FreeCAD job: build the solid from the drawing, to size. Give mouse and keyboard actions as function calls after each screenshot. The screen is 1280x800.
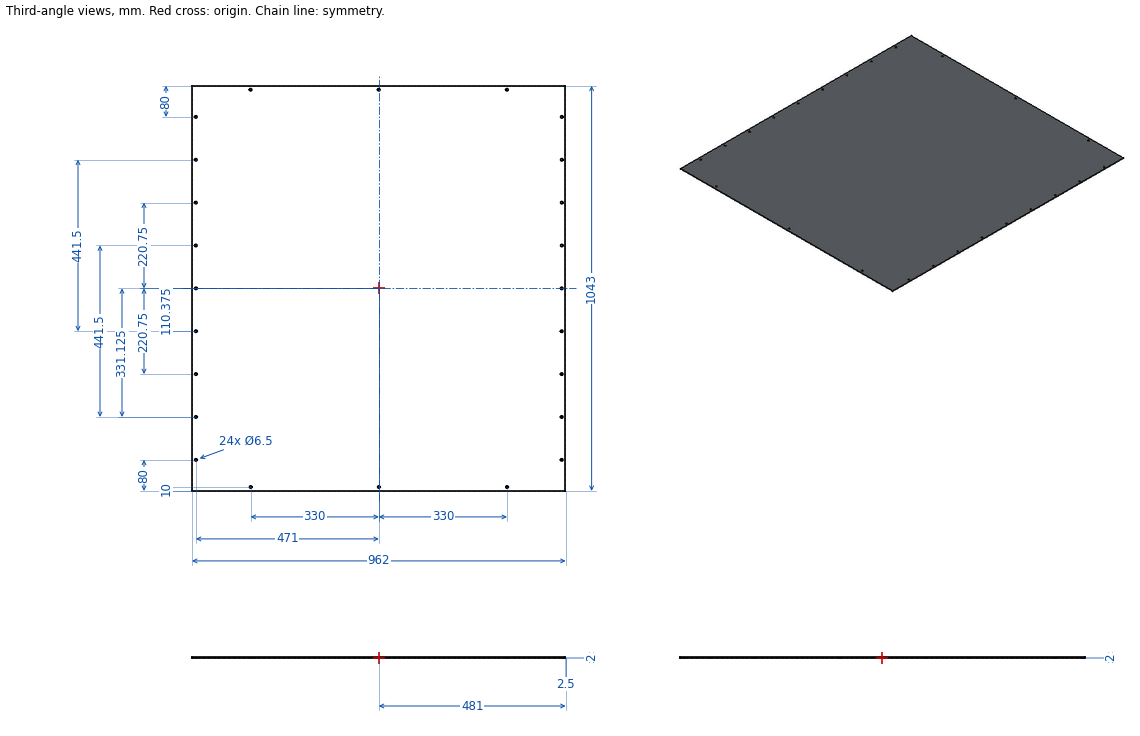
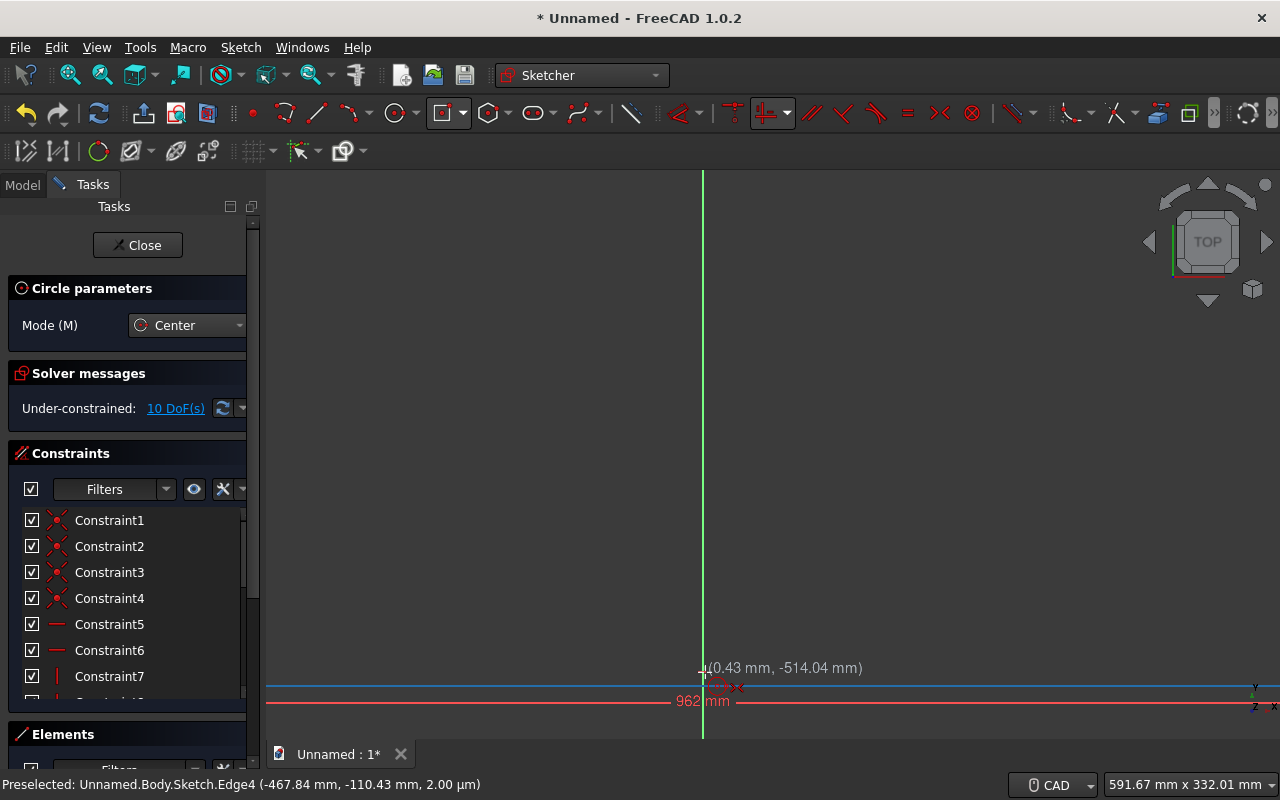
click(703, 669)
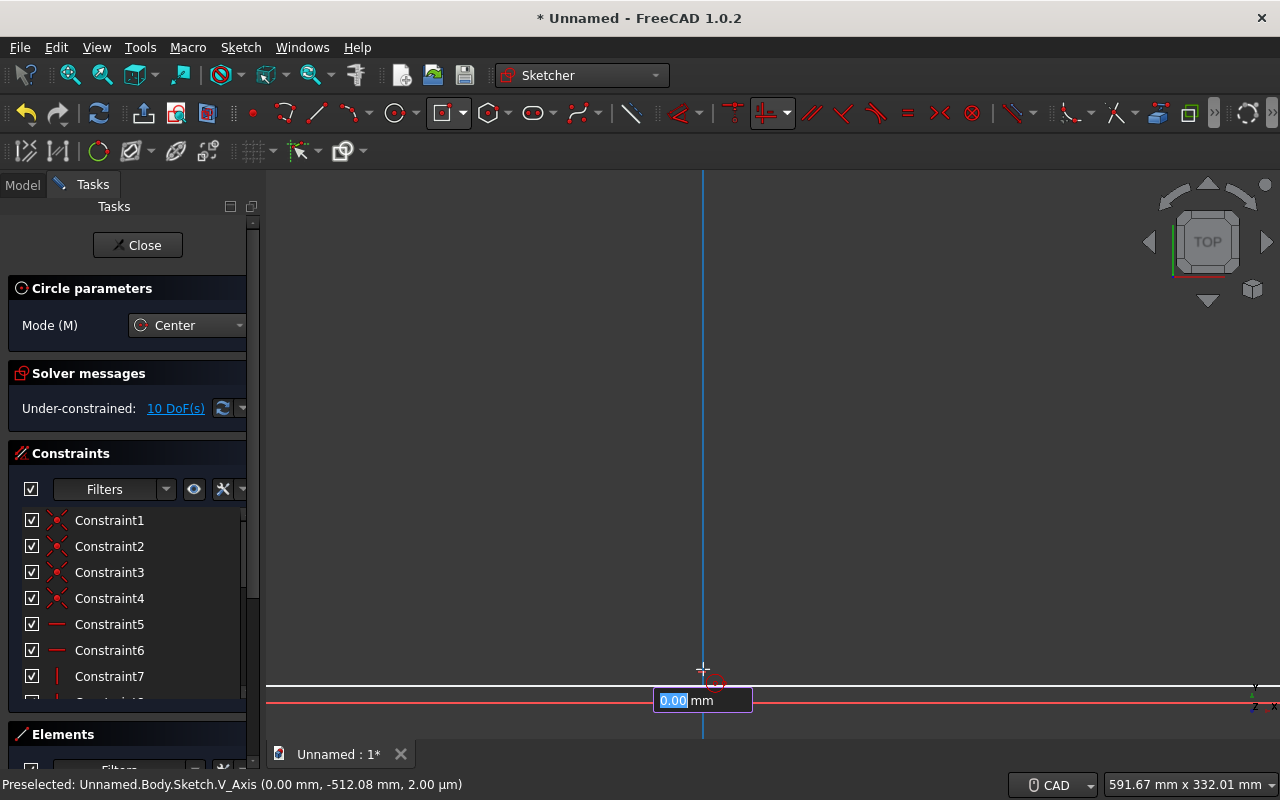
scroll(708, 667, up, 6)
move(708, 665)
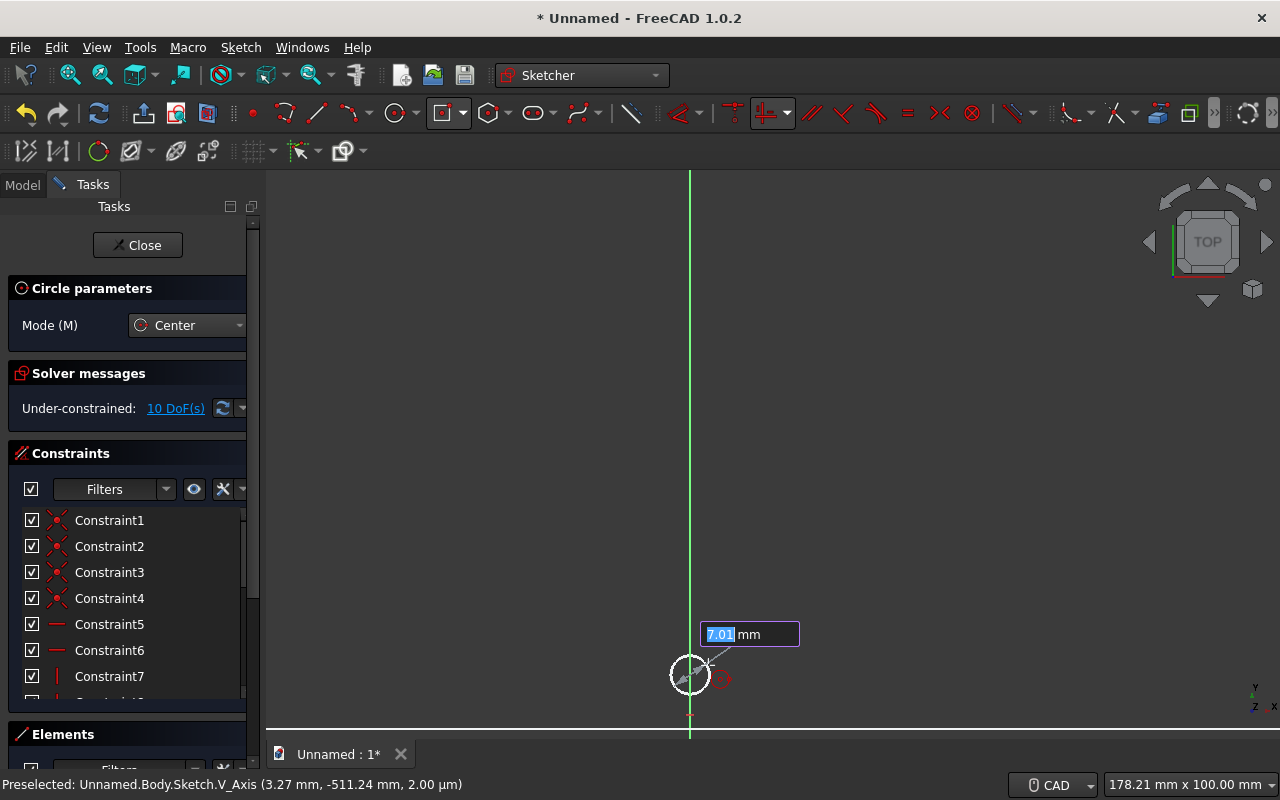
text(6.5)
key(Return)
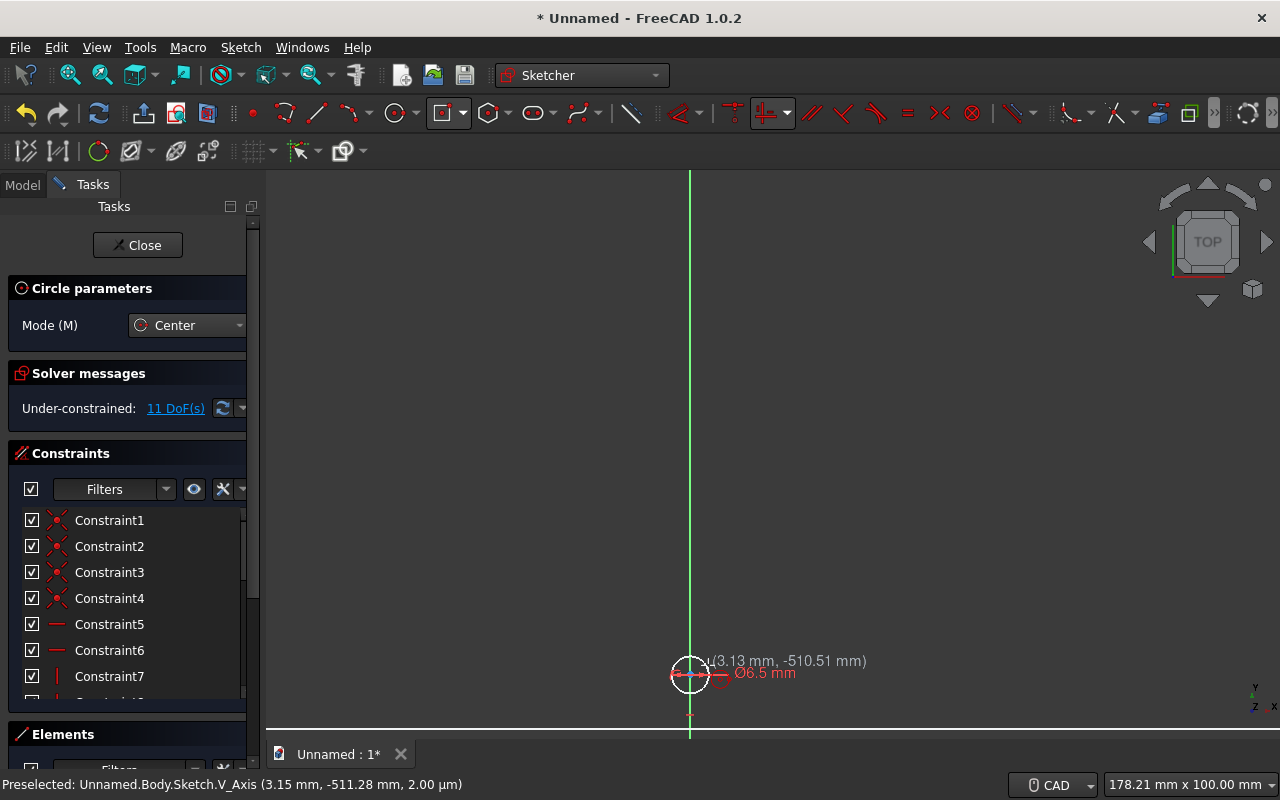
scroll(705, 629, down, 14)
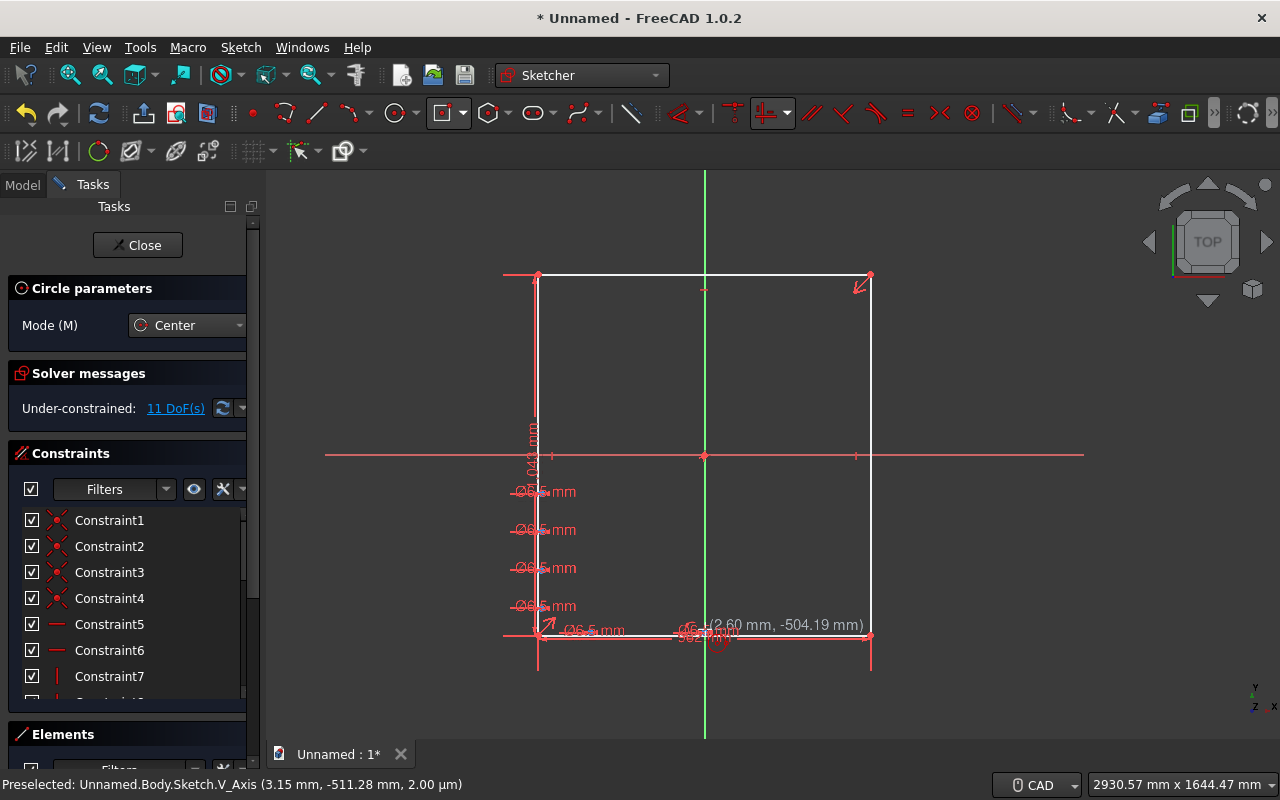
scroll(819, 632, up, 16)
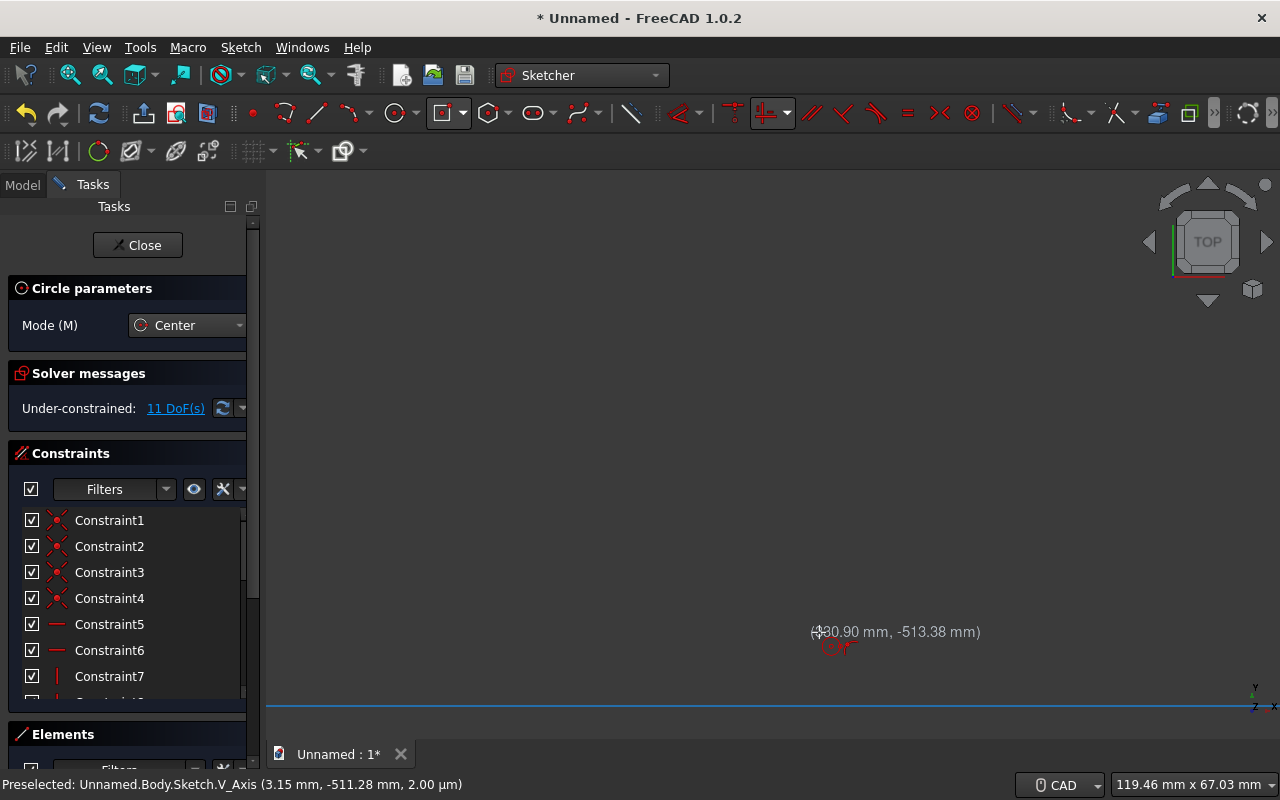
scroll(846, 673, down, 15)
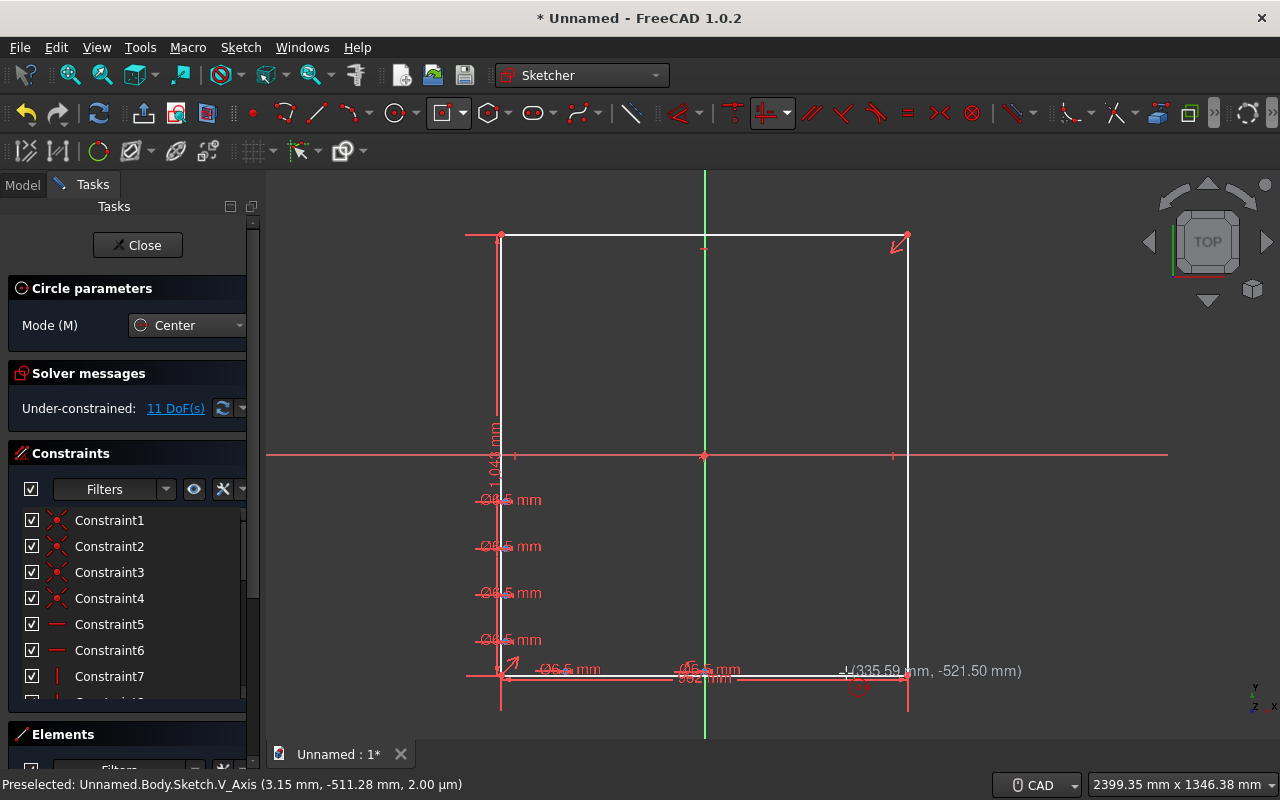
scroll(844, 671, up, 7)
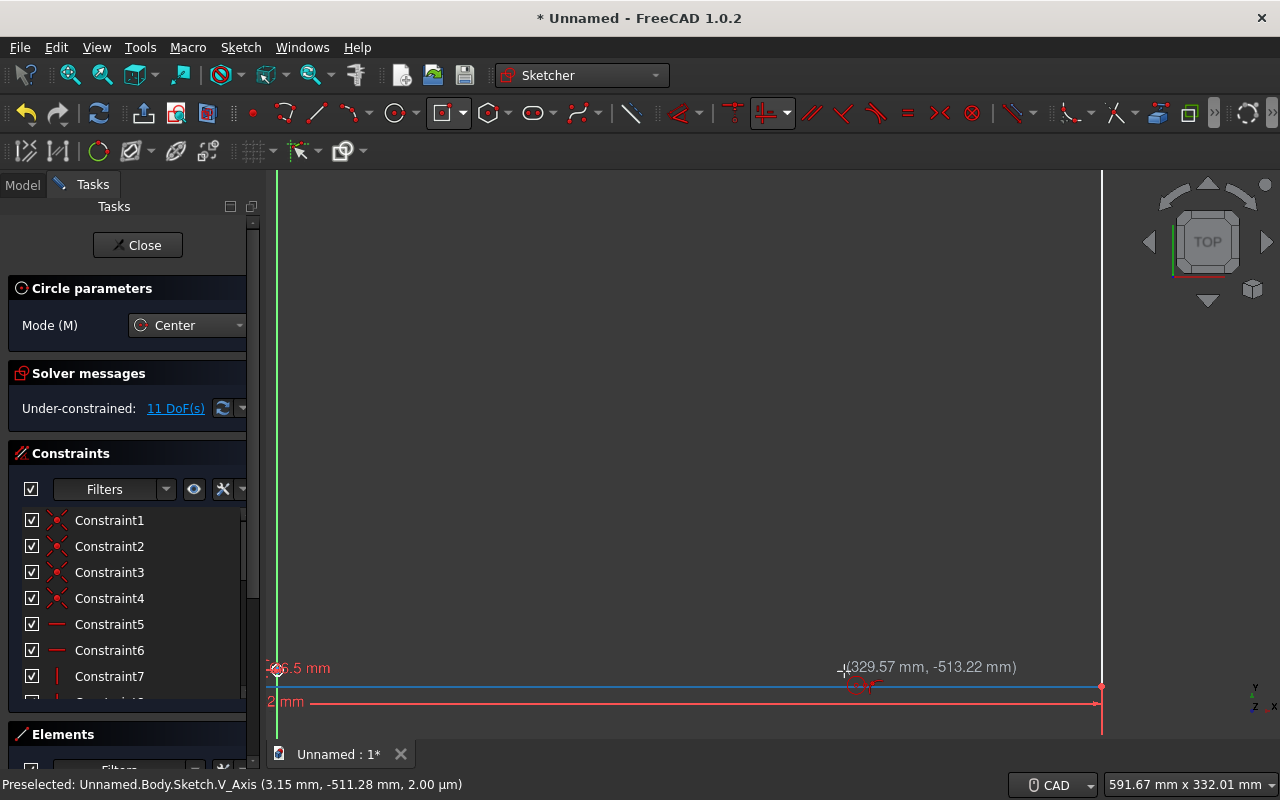
click(843, 669)
move(847, 665)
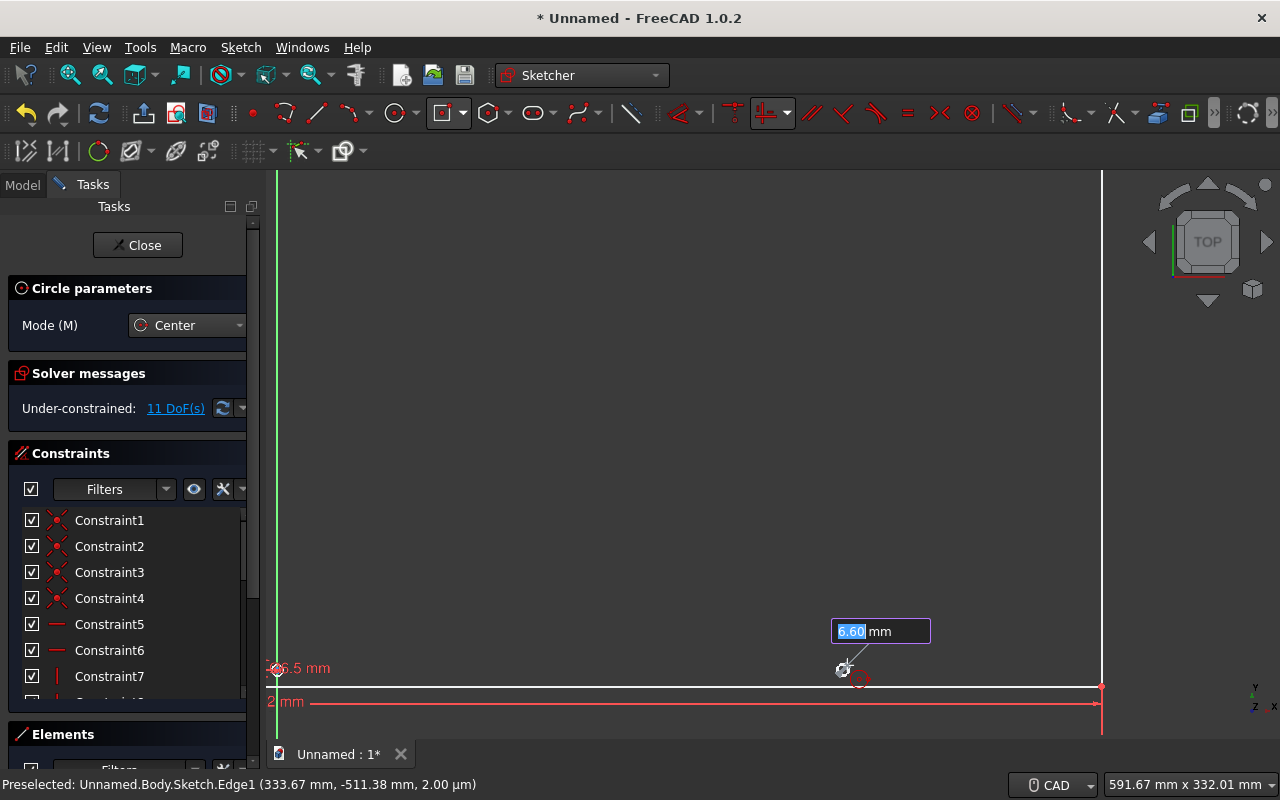
text(6.5)
key(Return)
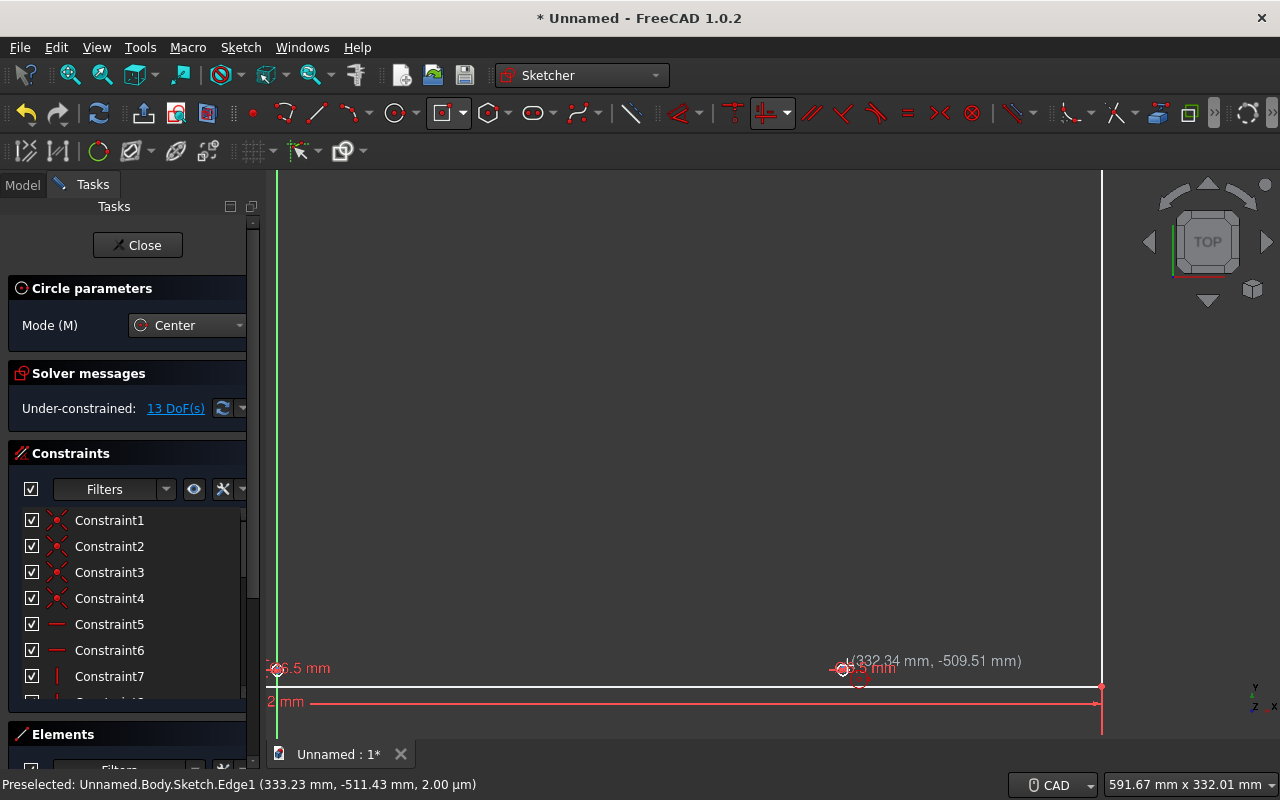
scroll(1085, 549, up, 8)